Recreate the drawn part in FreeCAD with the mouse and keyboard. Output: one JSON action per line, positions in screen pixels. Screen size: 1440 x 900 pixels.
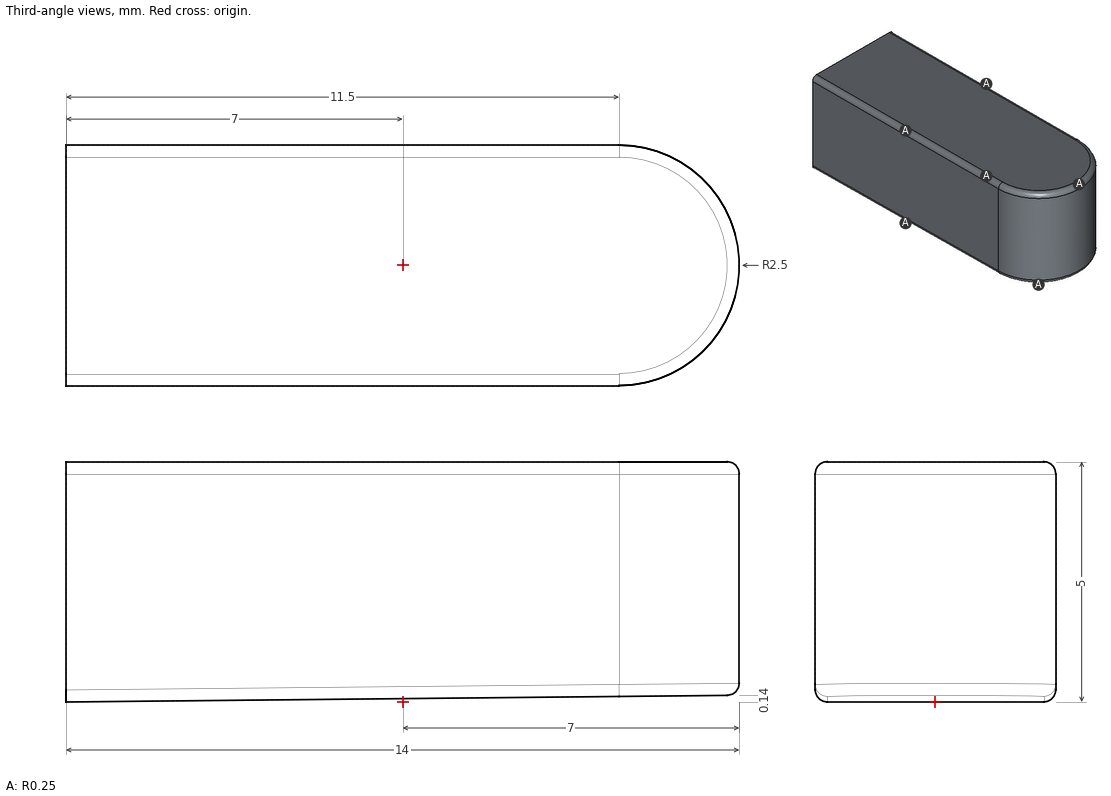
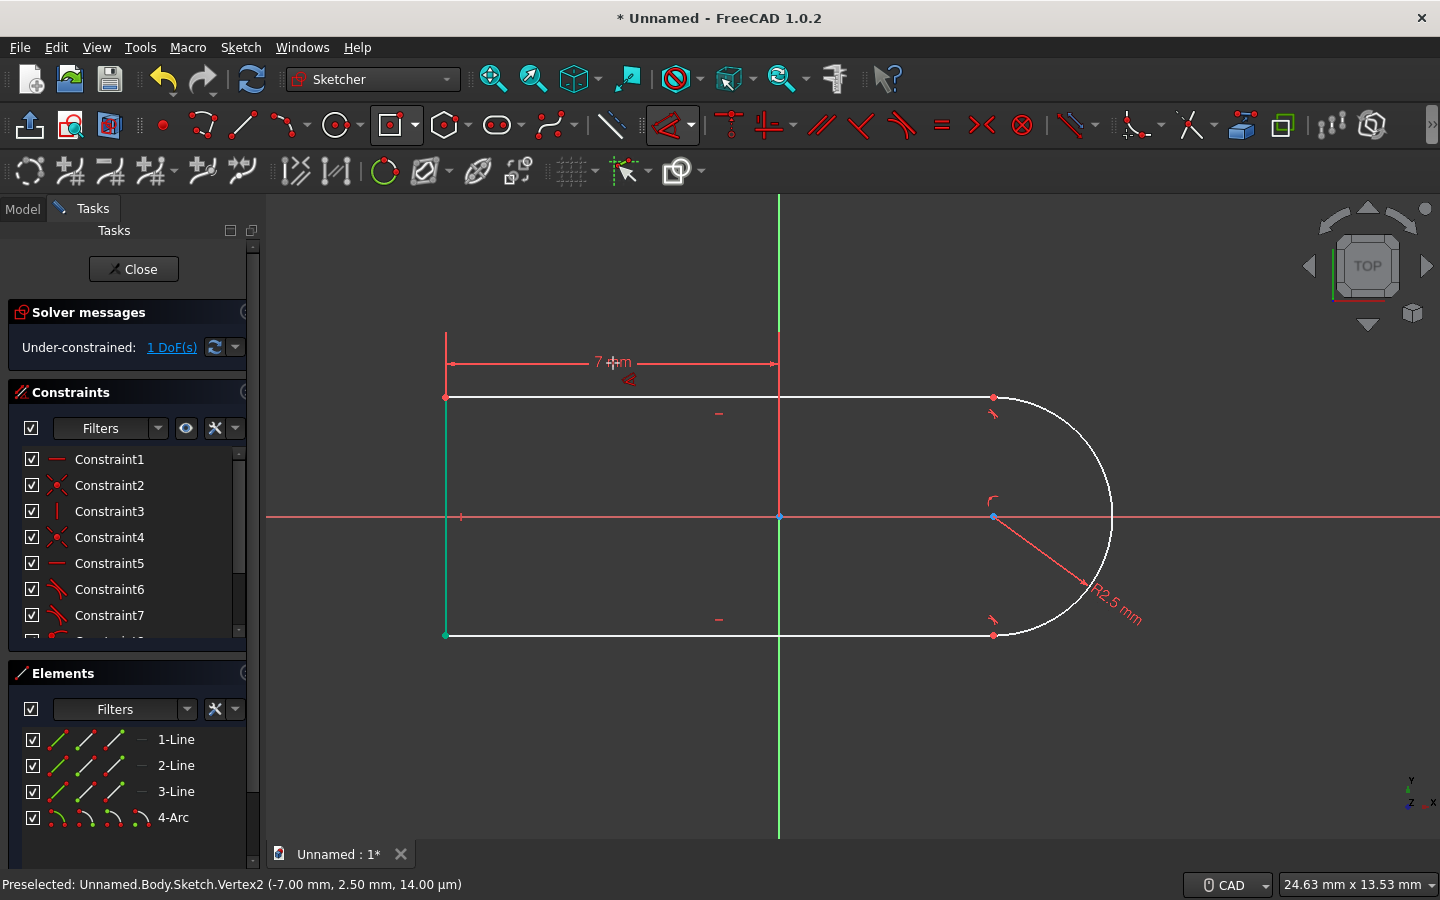
{"action": "left_click", "coordinate": [829, 397]}
{"action": "left_click", "coordinate": [720, 363]}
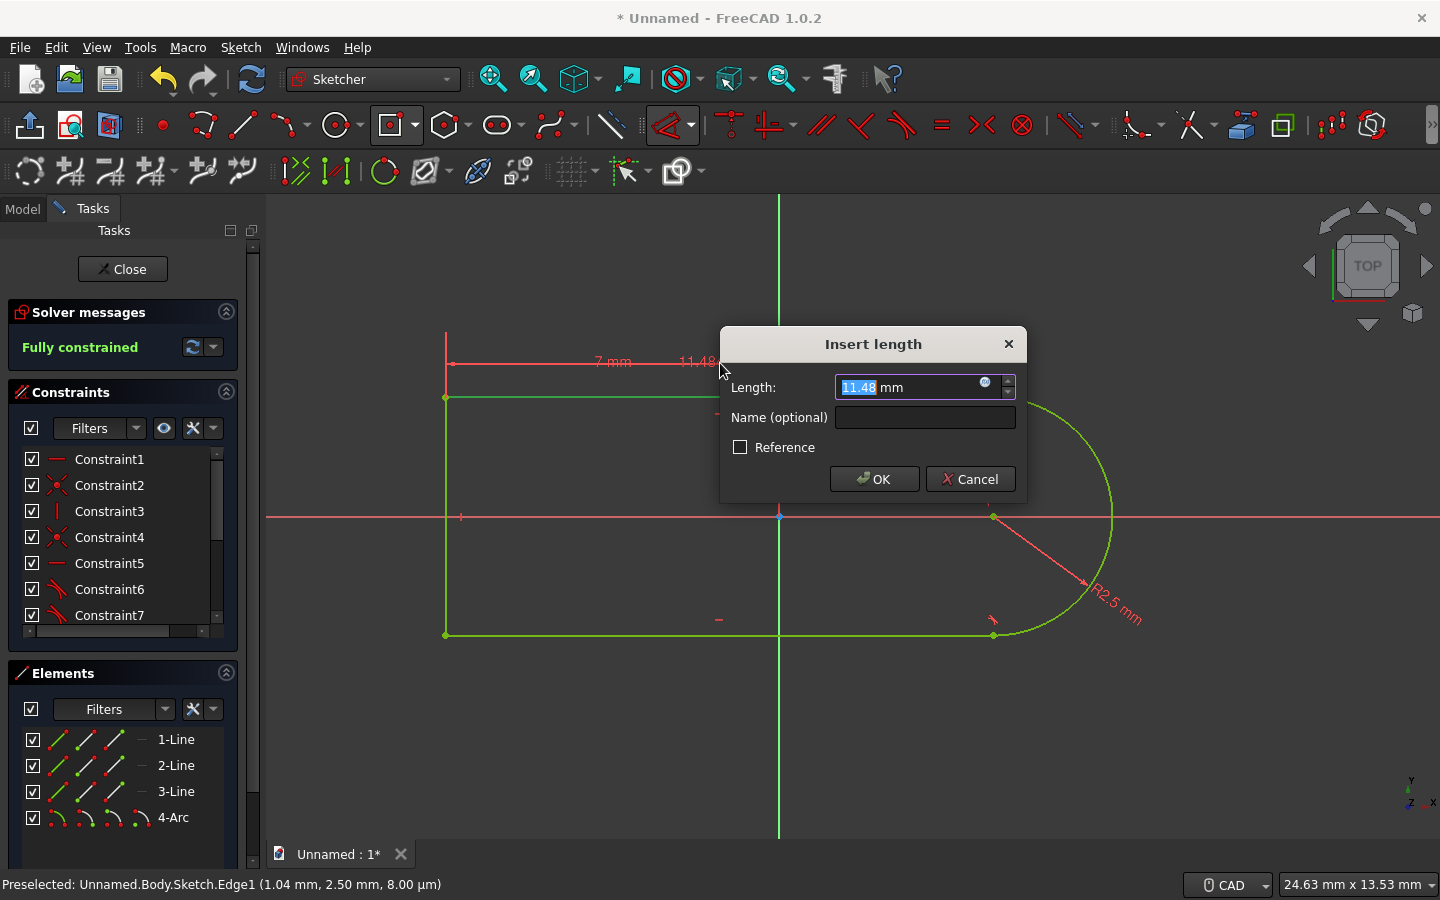
{"action": "type", "text": "11.5"}
{"action": "key", "text": "Return"}
{"action": "key", "text": "Escape"}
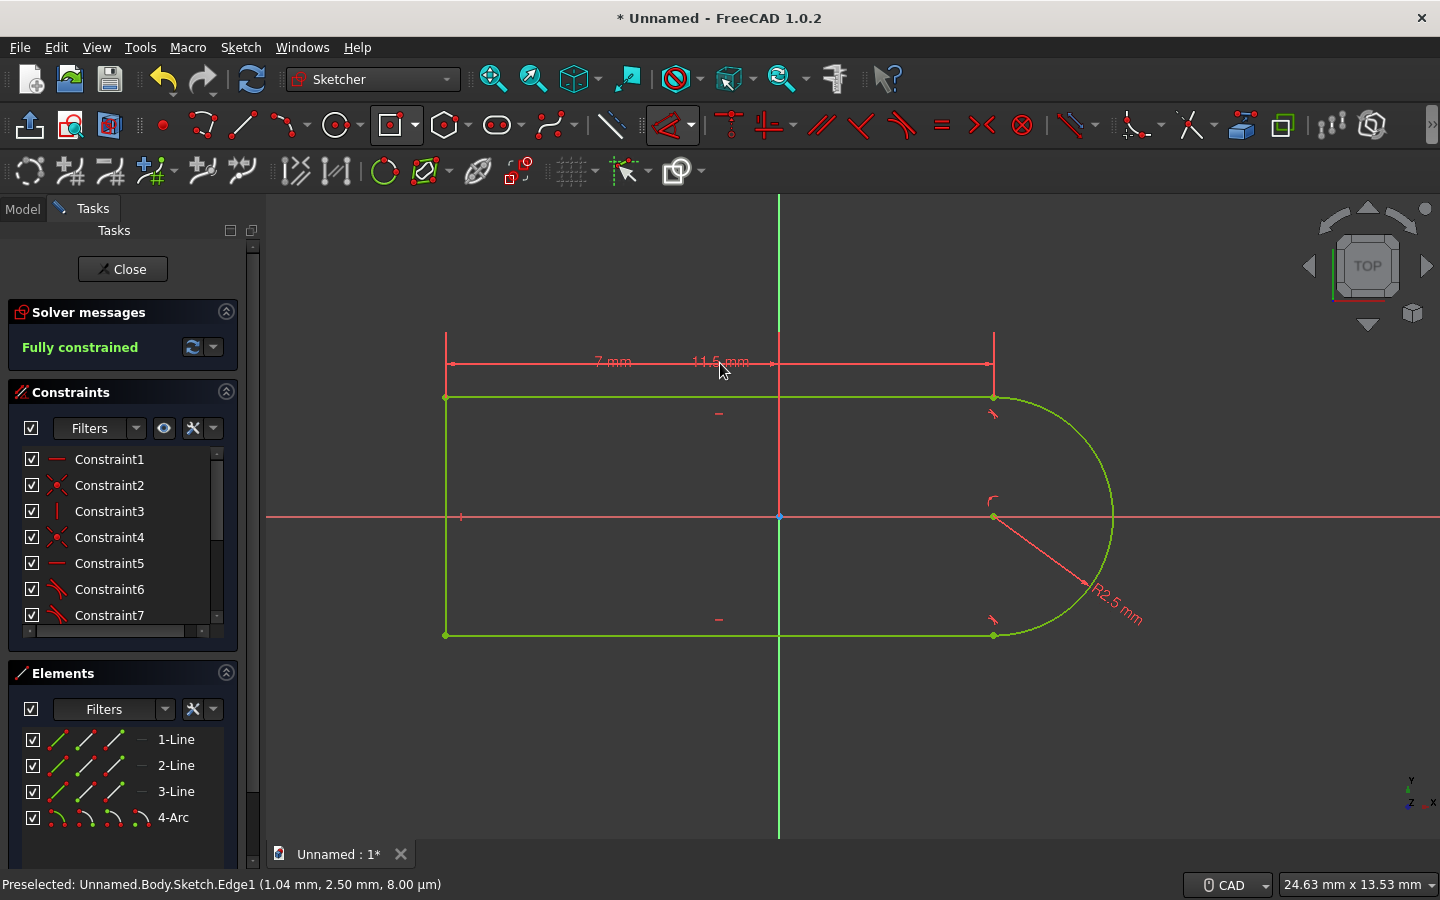
{"action": "left_click", "coordinate": [123, 269]}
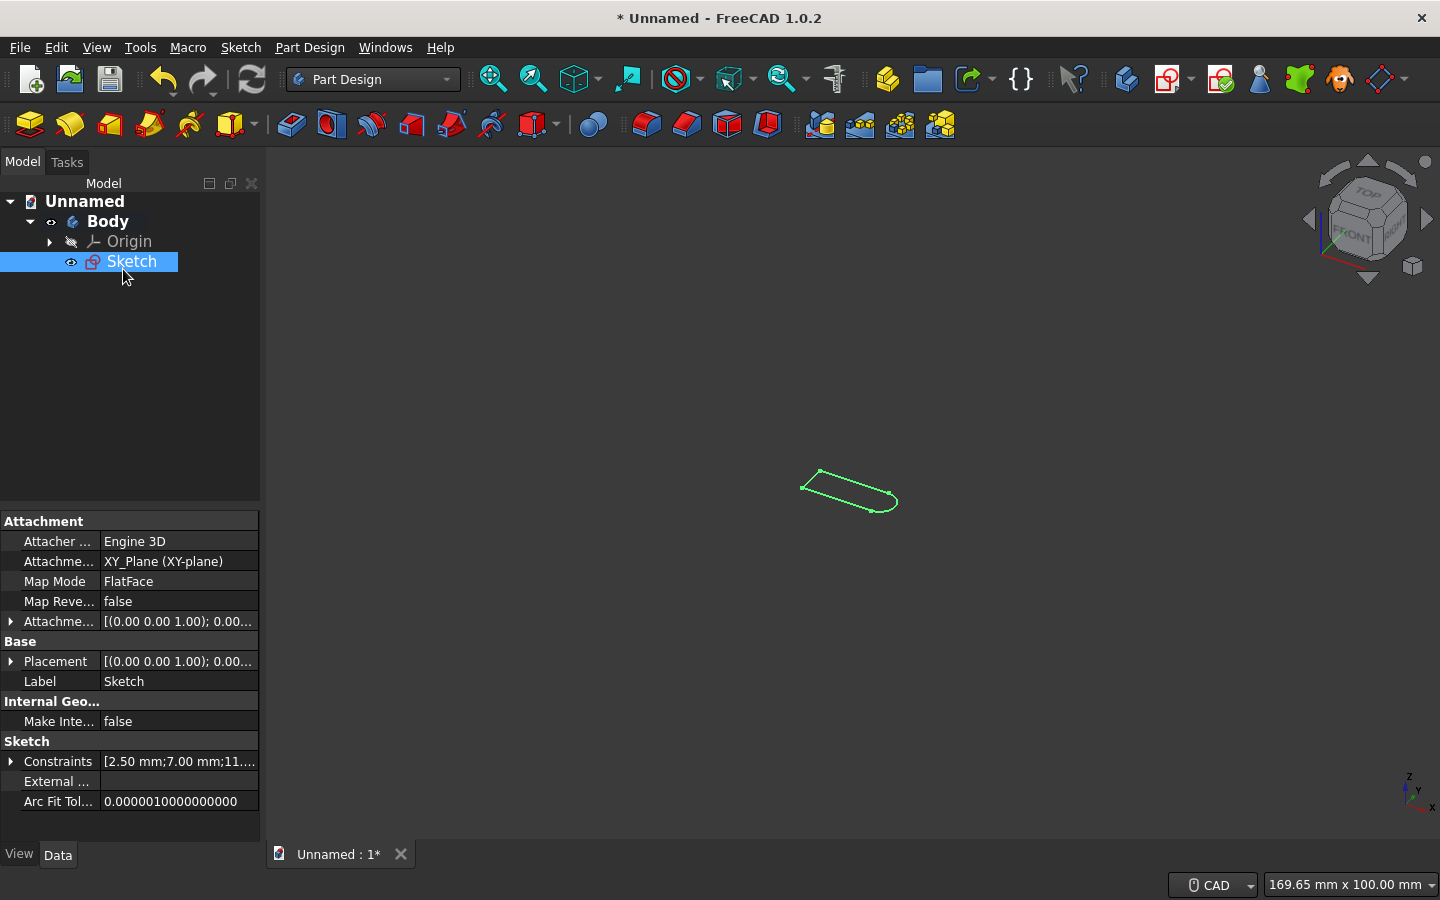
{"action": "left_click", "coordinate": [30, 124]}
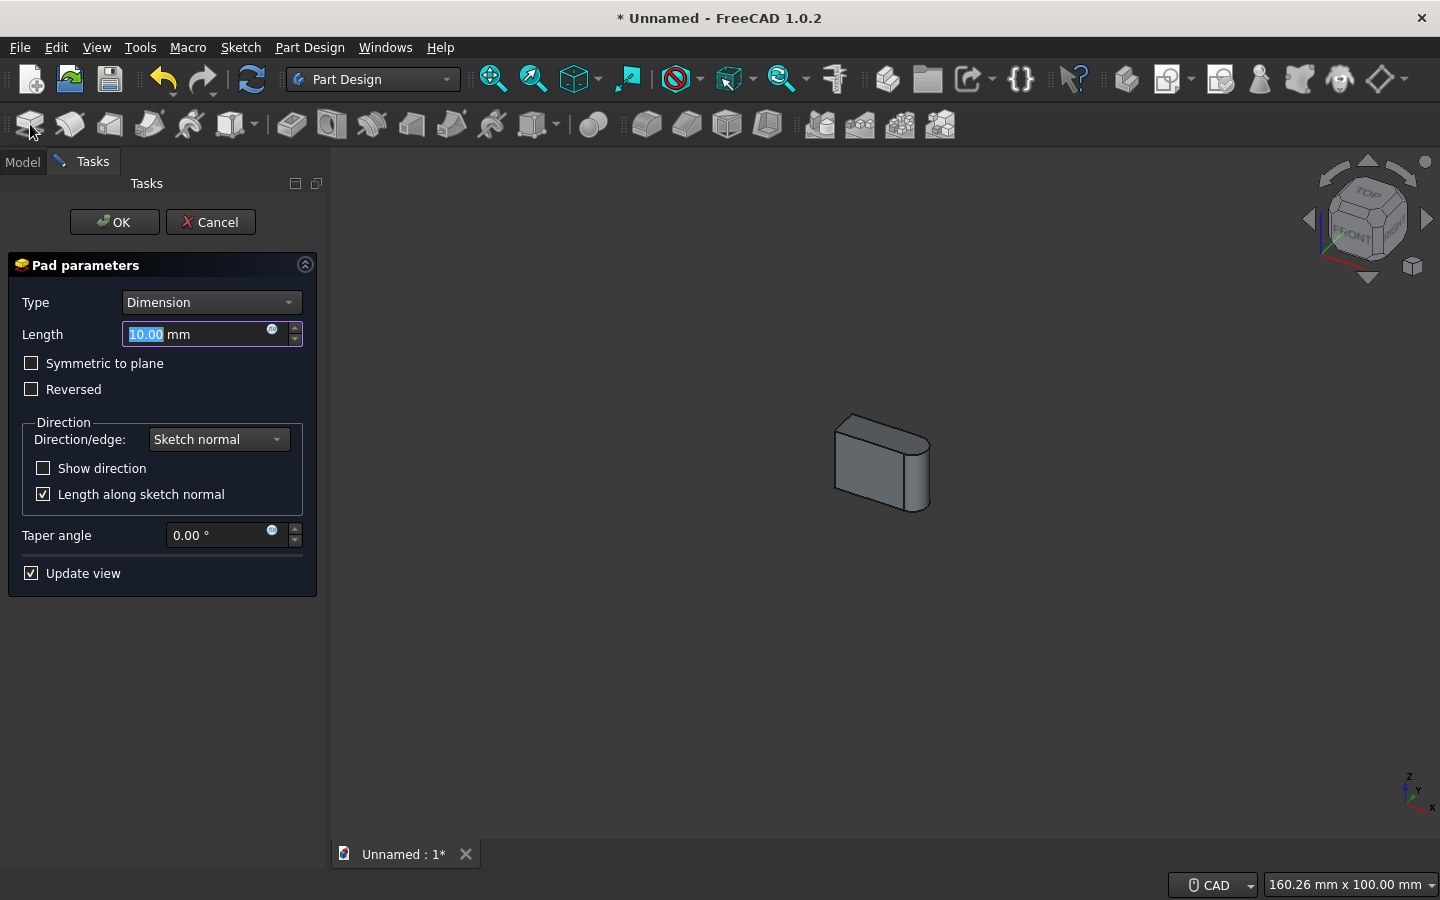
{"action": "type", "text": "5"}
{"action": "key", "text": "Tab"}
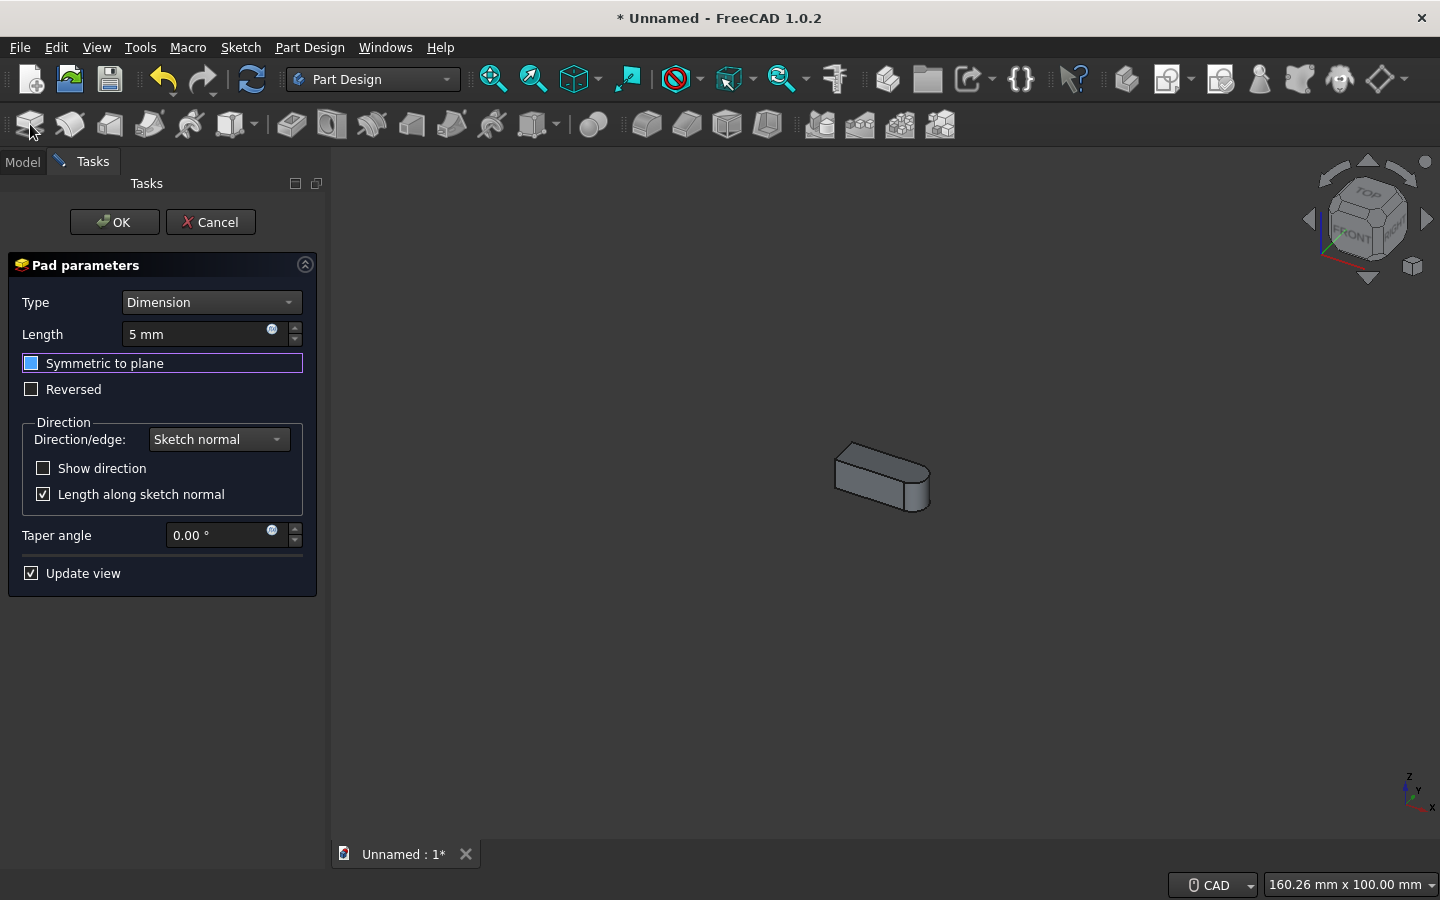
{"action": "left_click", "coordinate": [115, 222]}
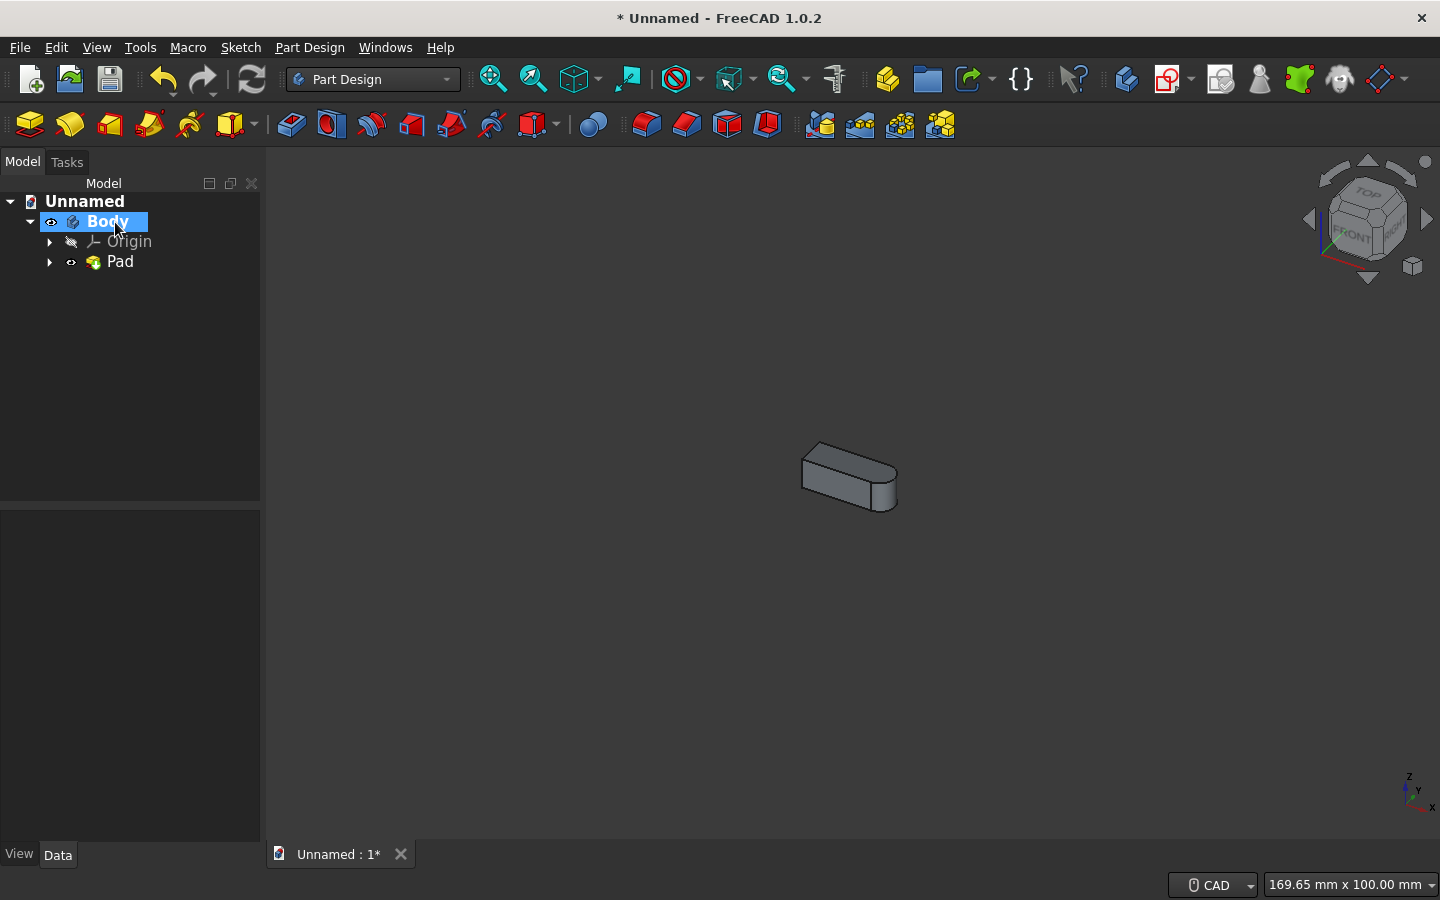
{"action": "key", "text": "v f"}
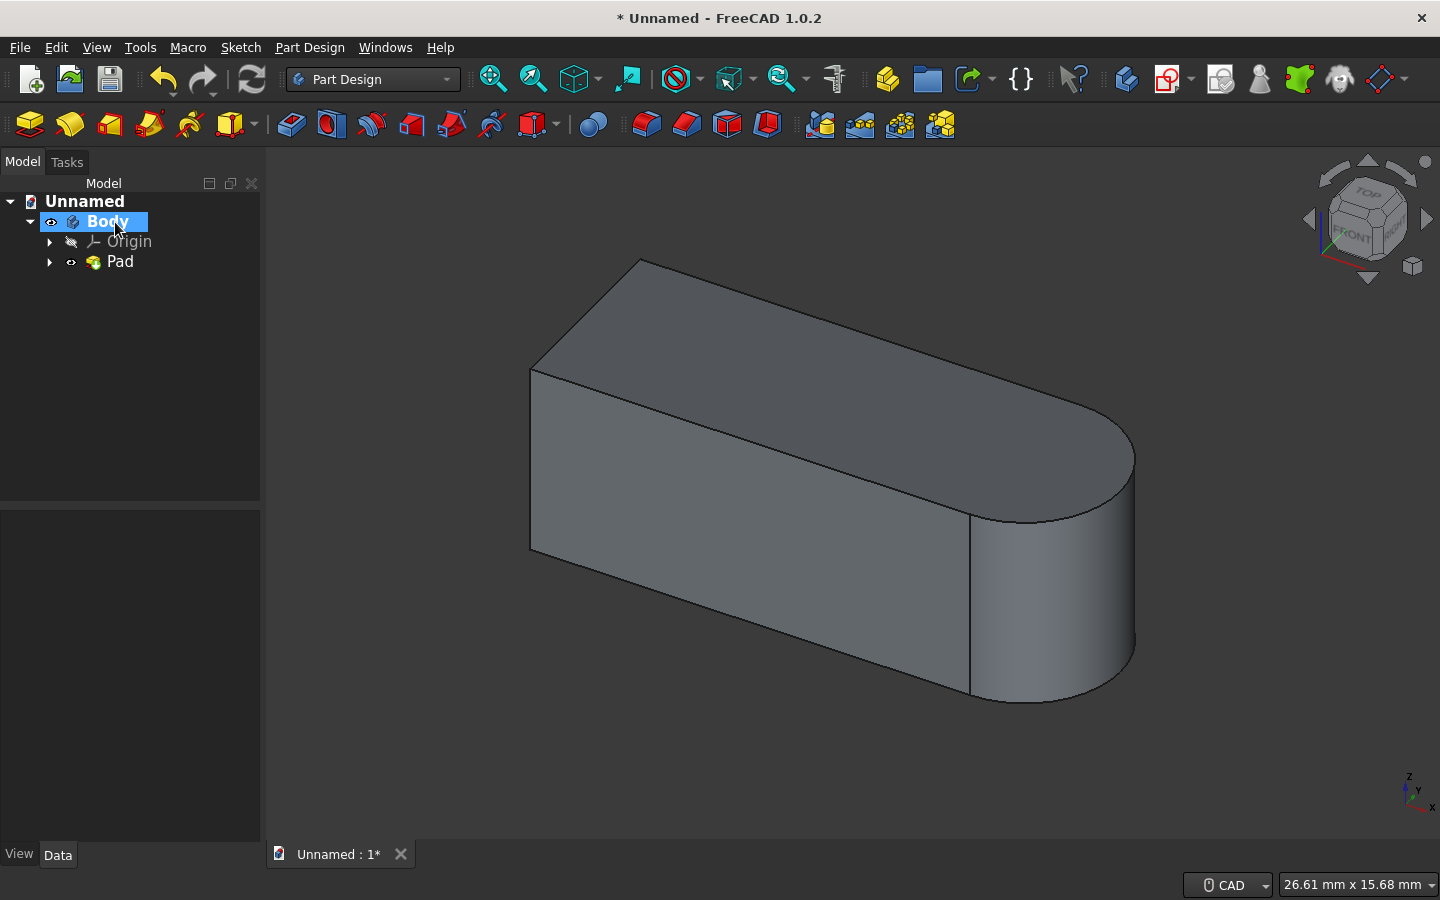
{"action": "left_click", "coordinate": [1168, 80]}